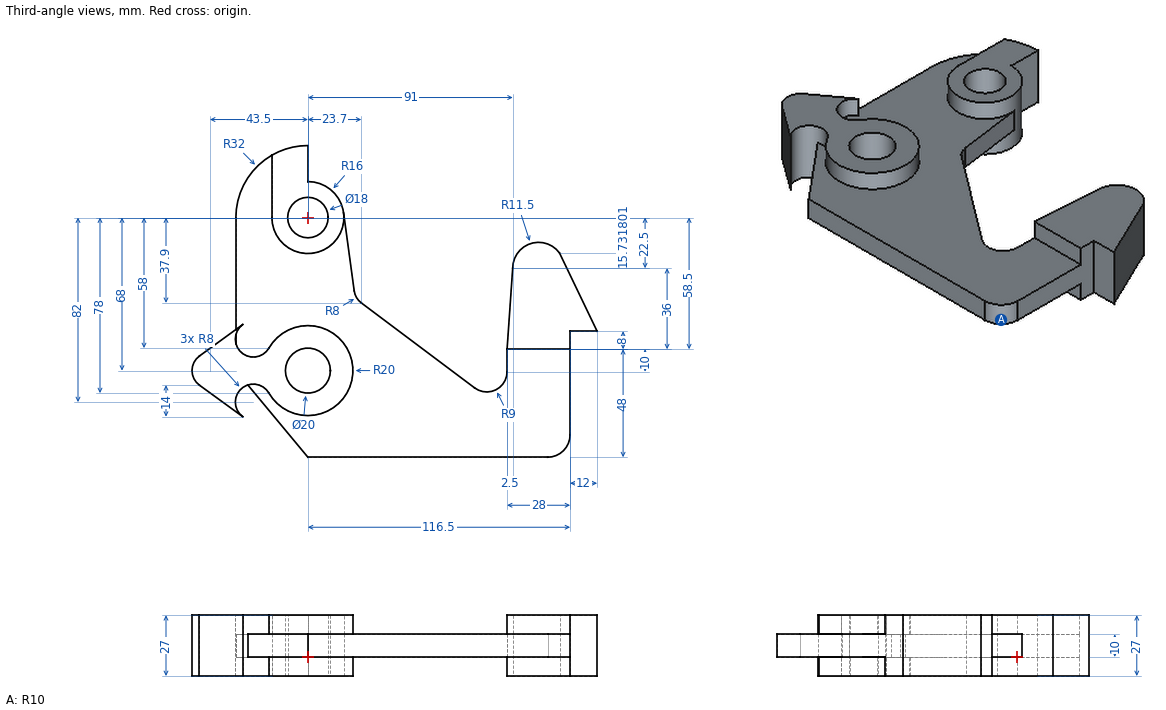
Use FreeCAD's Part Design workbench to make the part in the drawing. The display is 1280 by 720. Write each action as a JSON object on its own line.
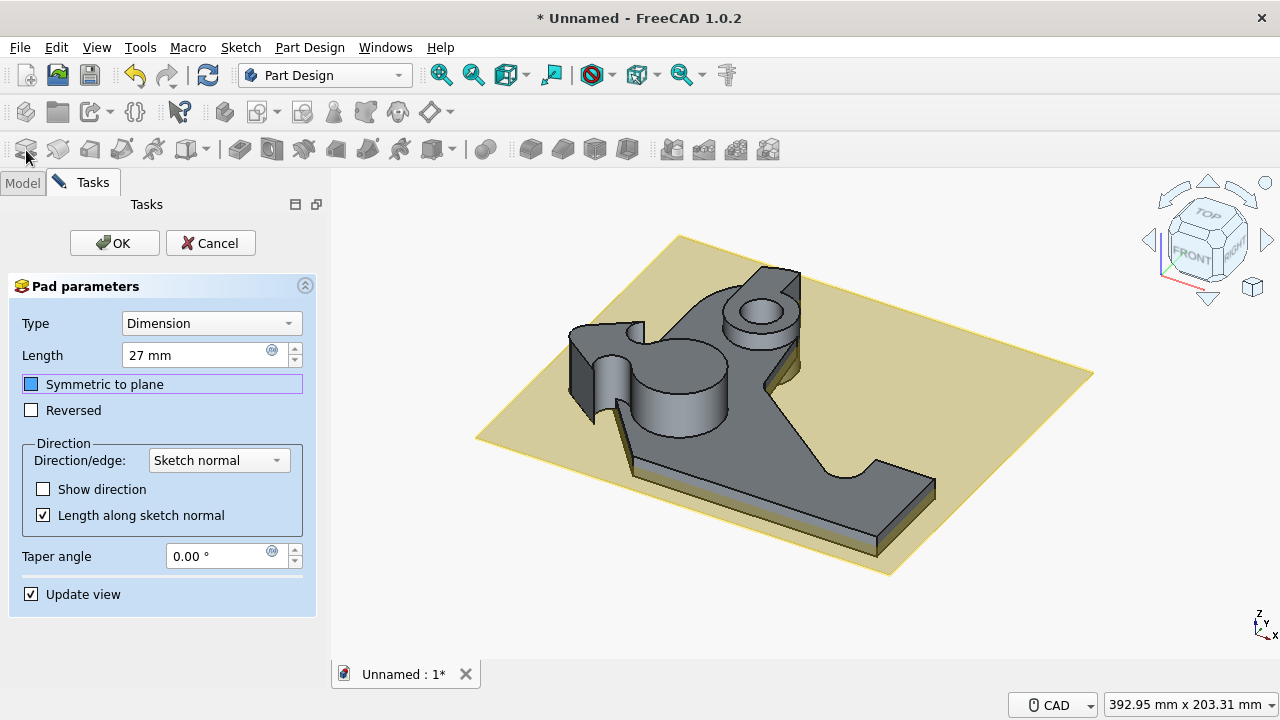
{"action": "left_click", "coordinate": [30, 384]}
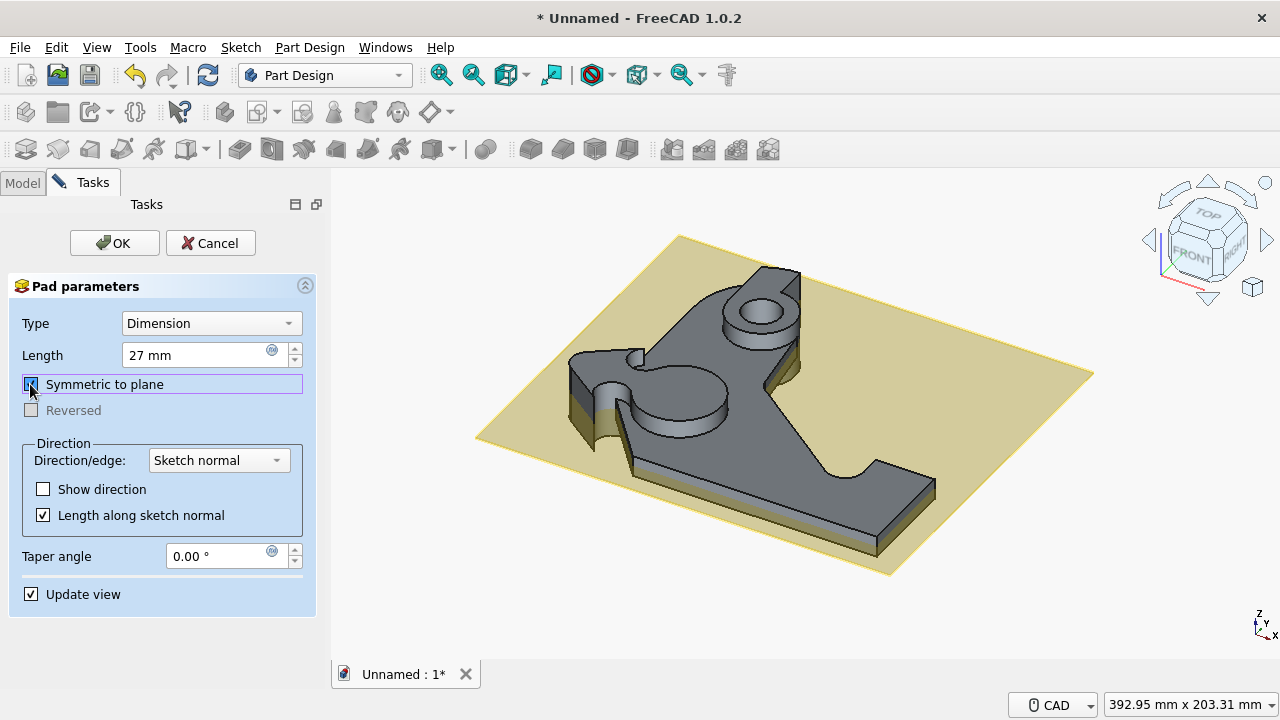
{"action": "left_click", "coordinate": [115, 243]}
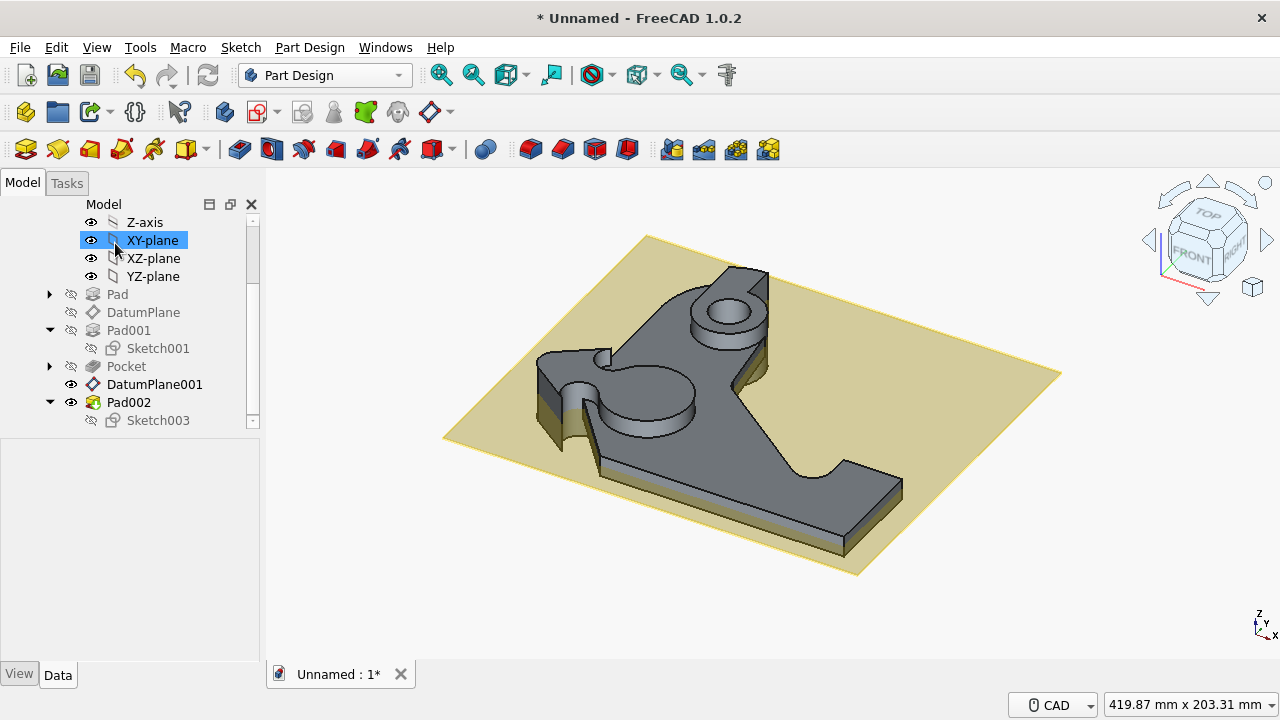
{"action": "left_click", "coordinate": [116, 384]}
{"action": "key", "text": "space"}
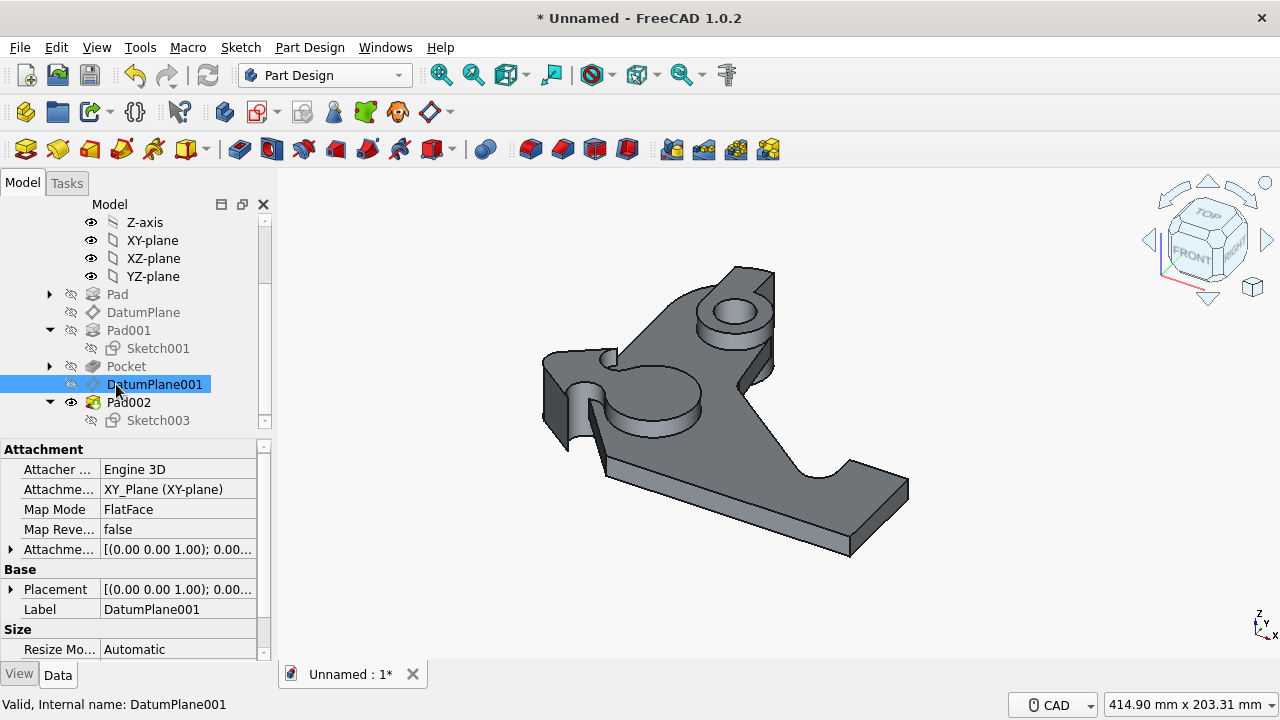
{"action": "left_click", "coordinate": [641, 388]}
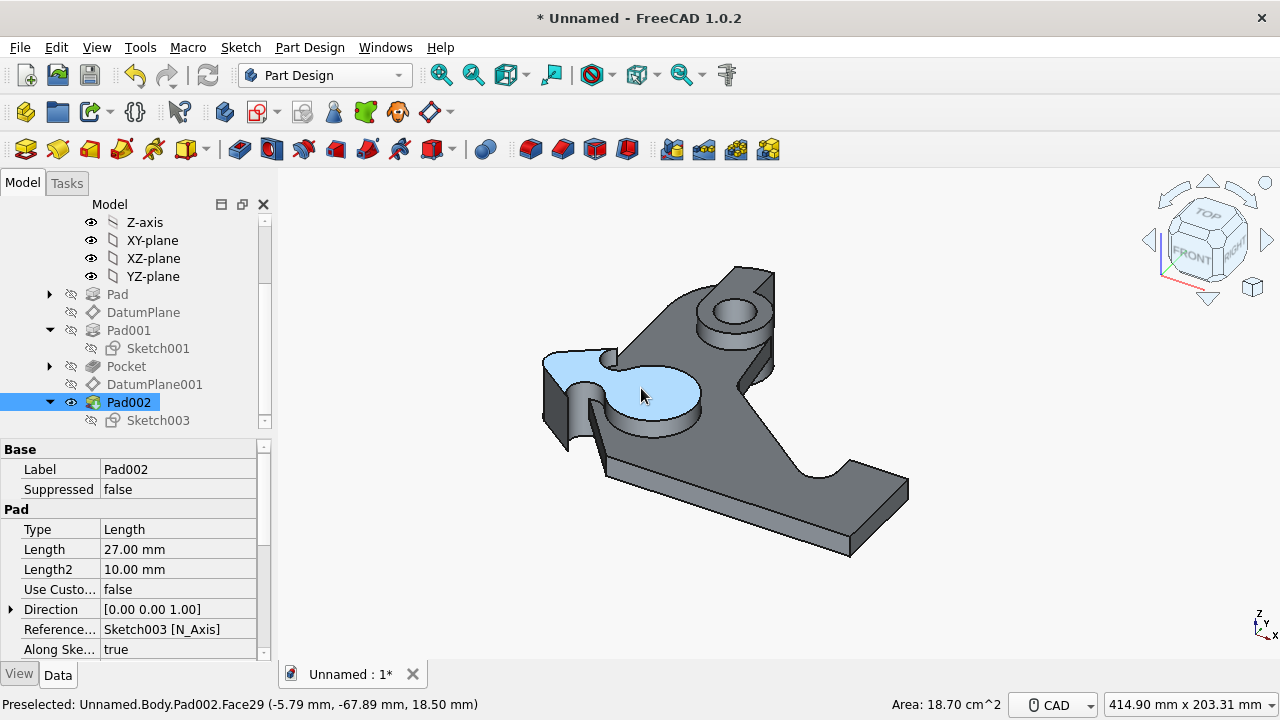
{"action": "left_click", "coordinate": [258, 112]}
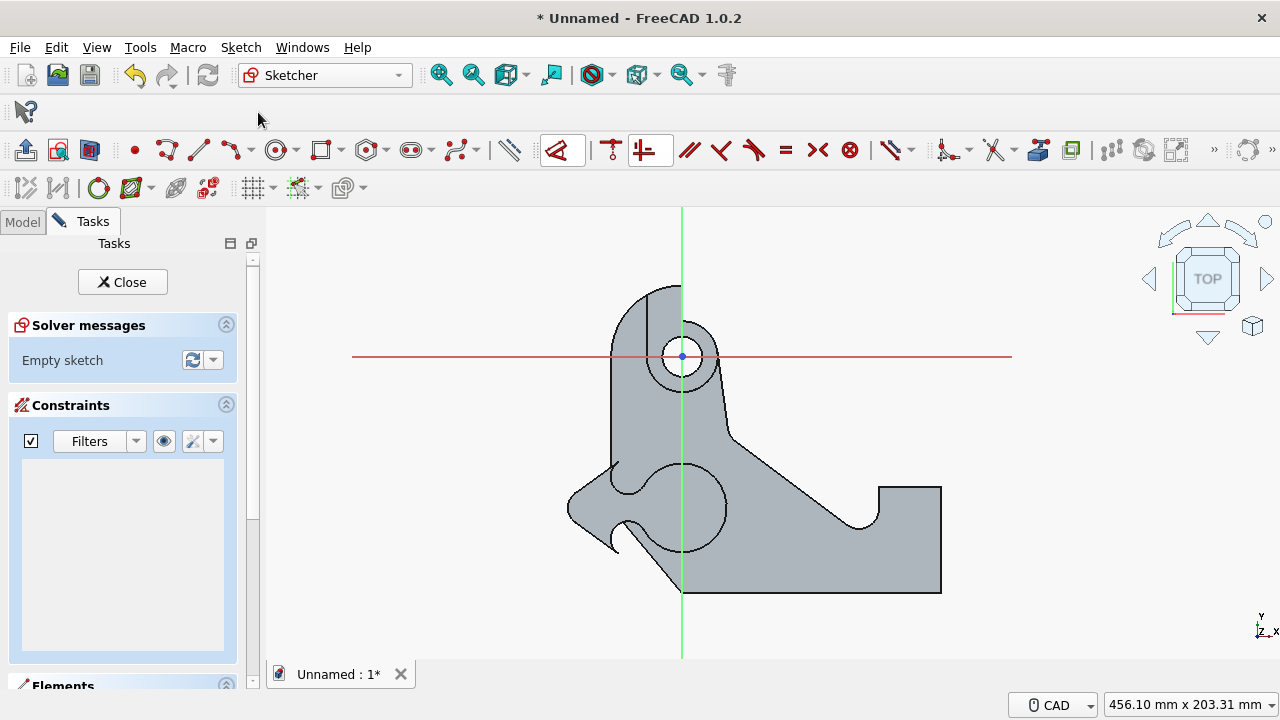
{"action": "scroll", "coordinate": [678, 523], "scroll_direction": "up", "scroll_amount": 9}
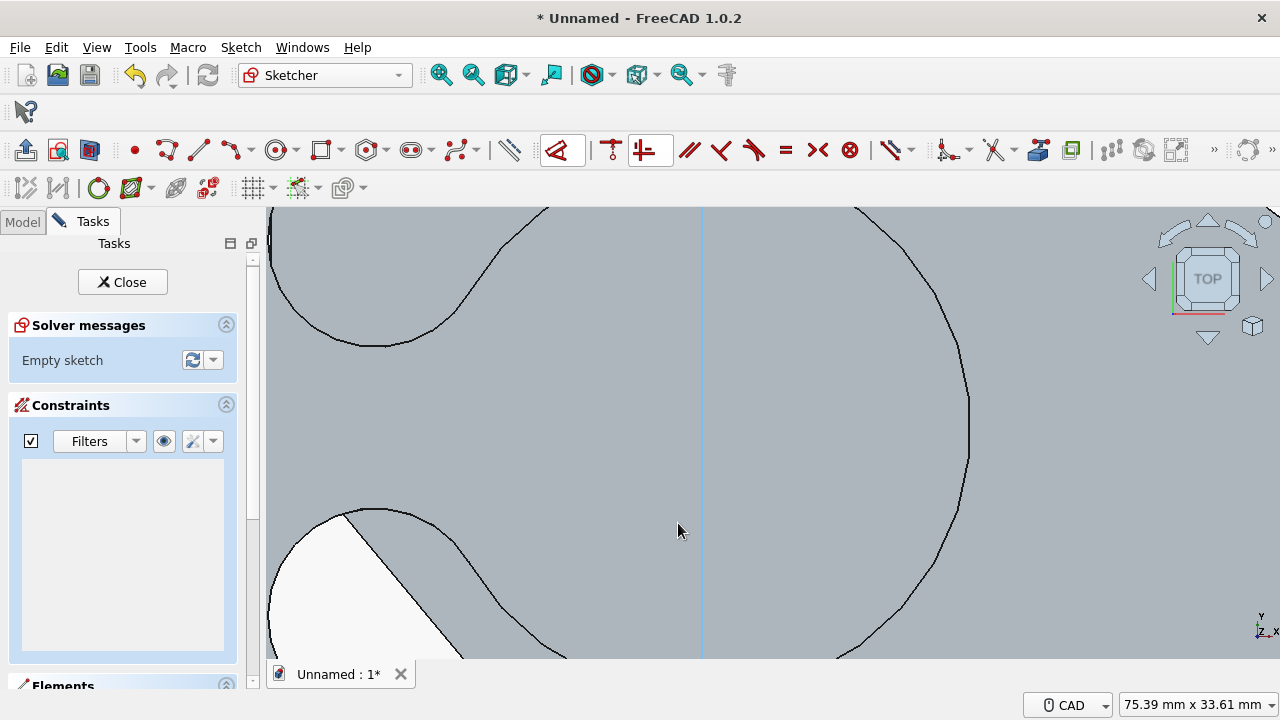
{"action": "left_click", "coordinate": [276, 150]}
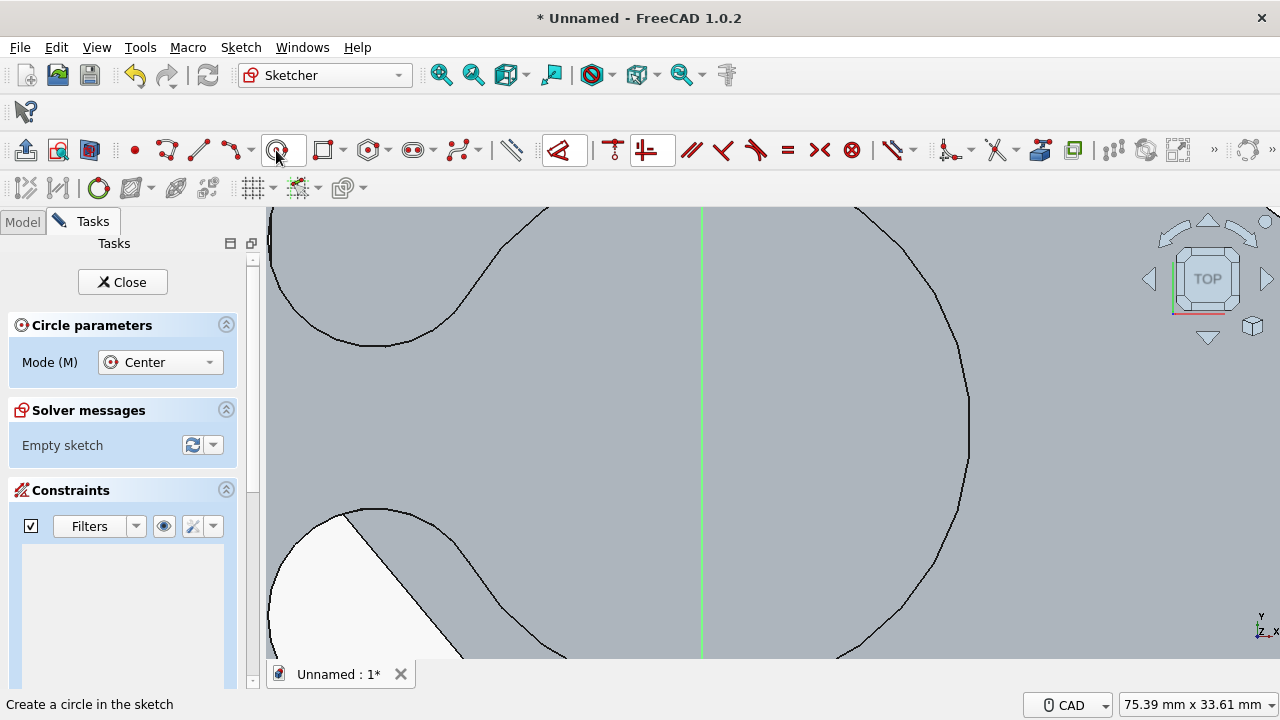
{"action": "left_click", "coordinate": [702, 428]}
{"action": "mouse_move", "coordinate": [797, 333]}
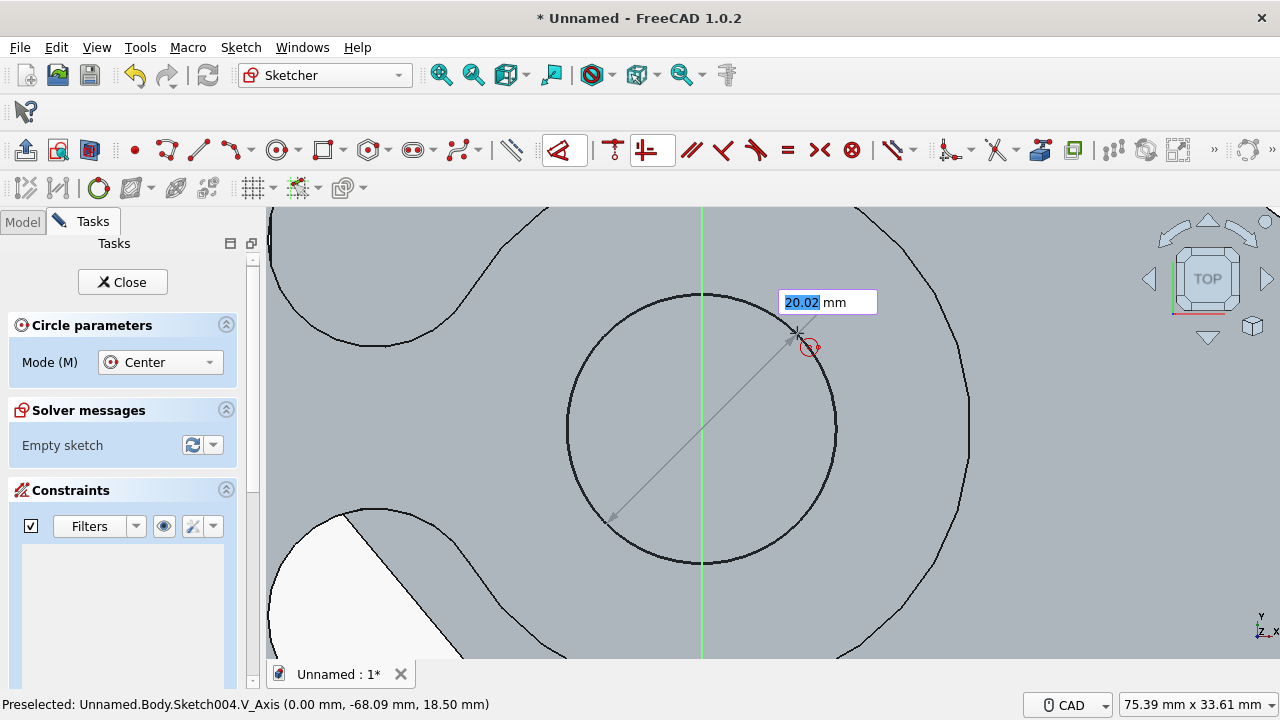
{"action": "type", "text": "20"}
{"action": "key", "text": "Return"}
{"action": "key", "text": "Escape"}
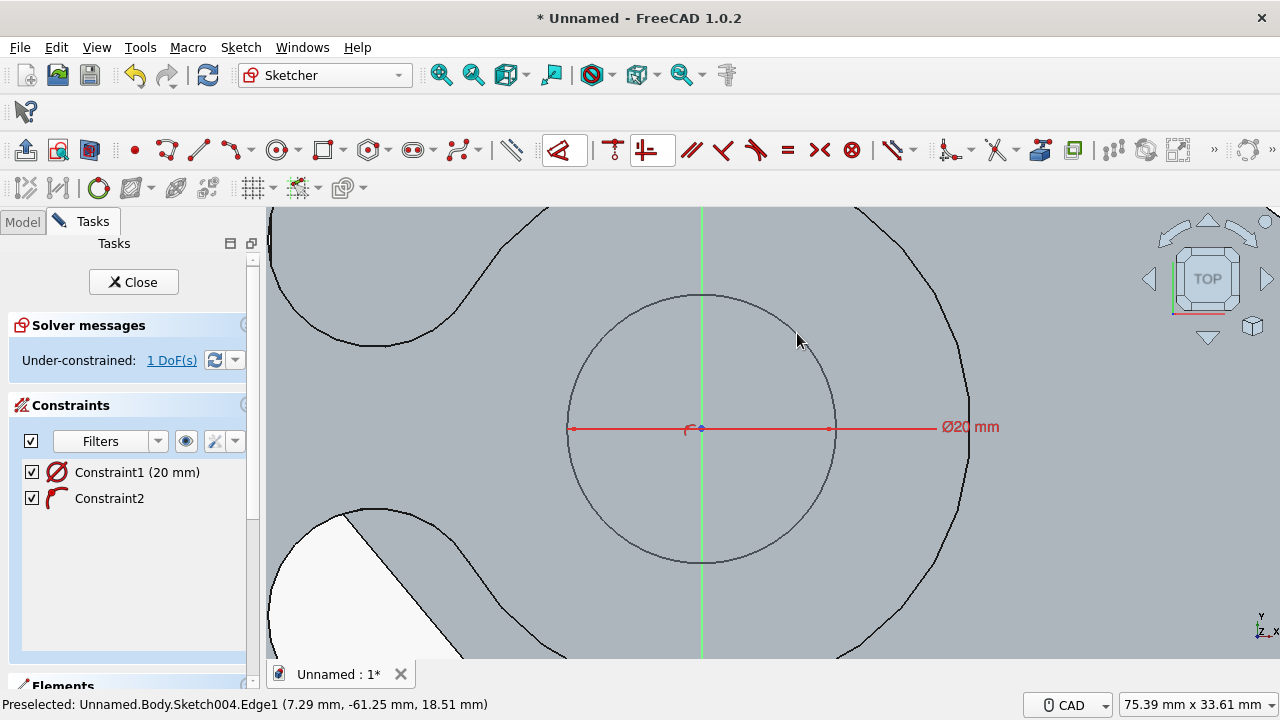
{"action": "left_click", "coordinate": [702, 429]}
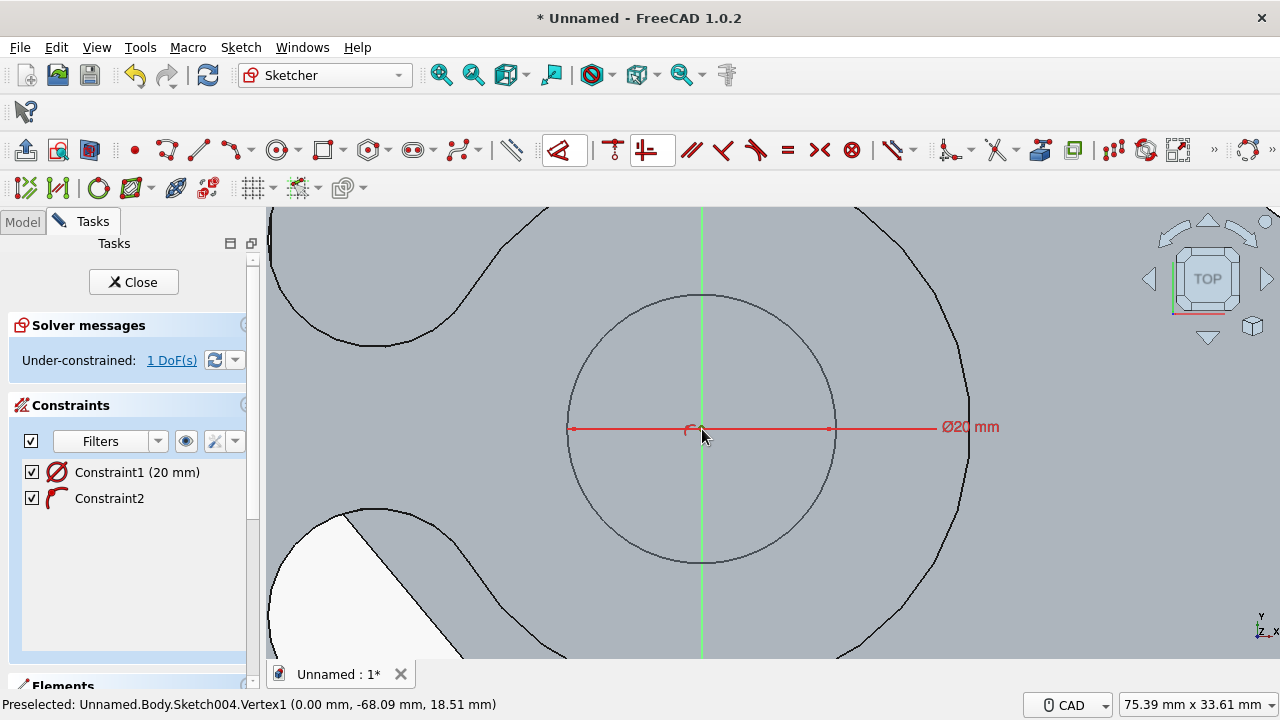
{"action": "key", "text": "i"}